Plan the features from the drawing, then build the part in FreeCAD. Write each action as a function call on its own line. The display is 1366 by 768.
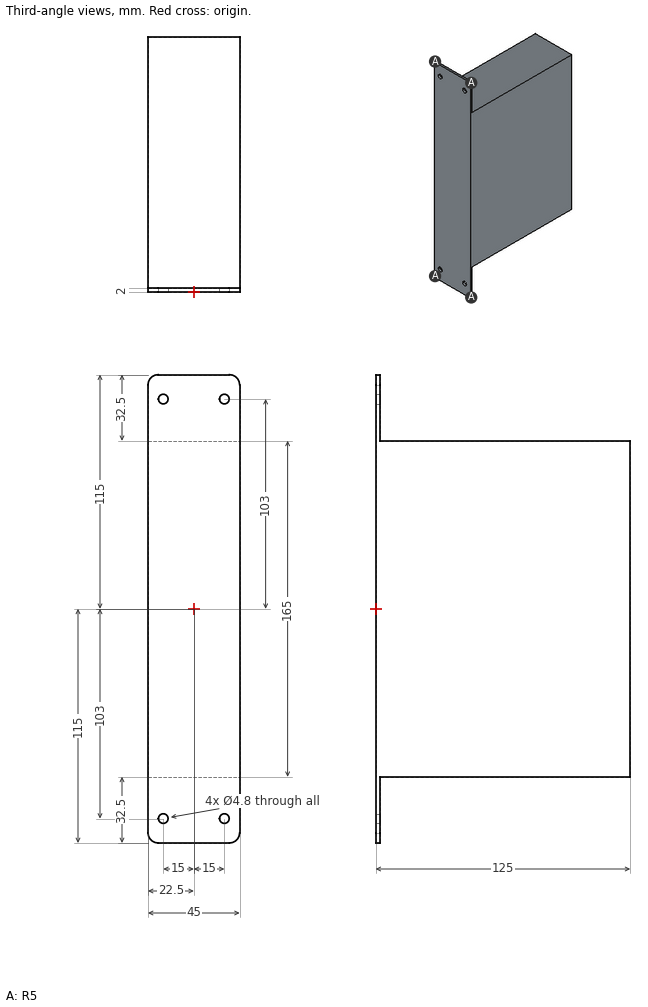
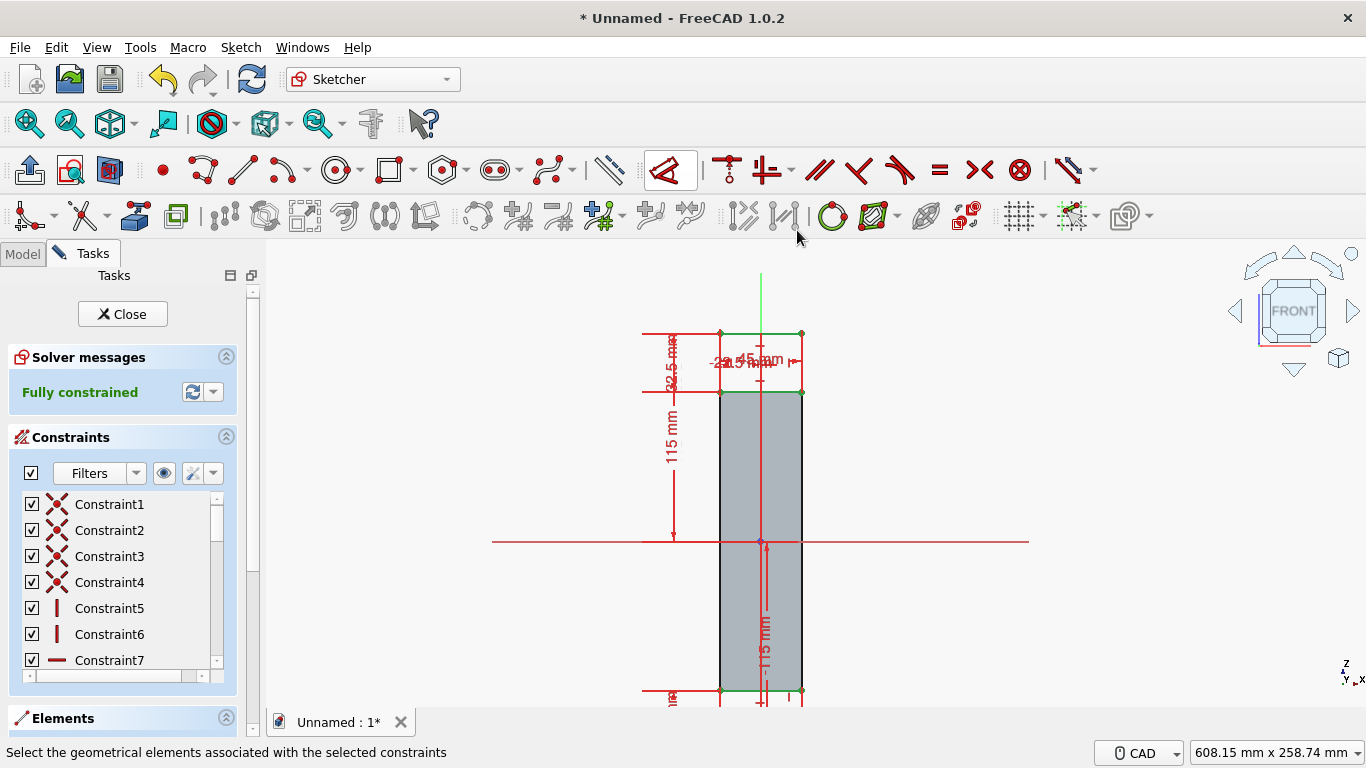
click(123, 314)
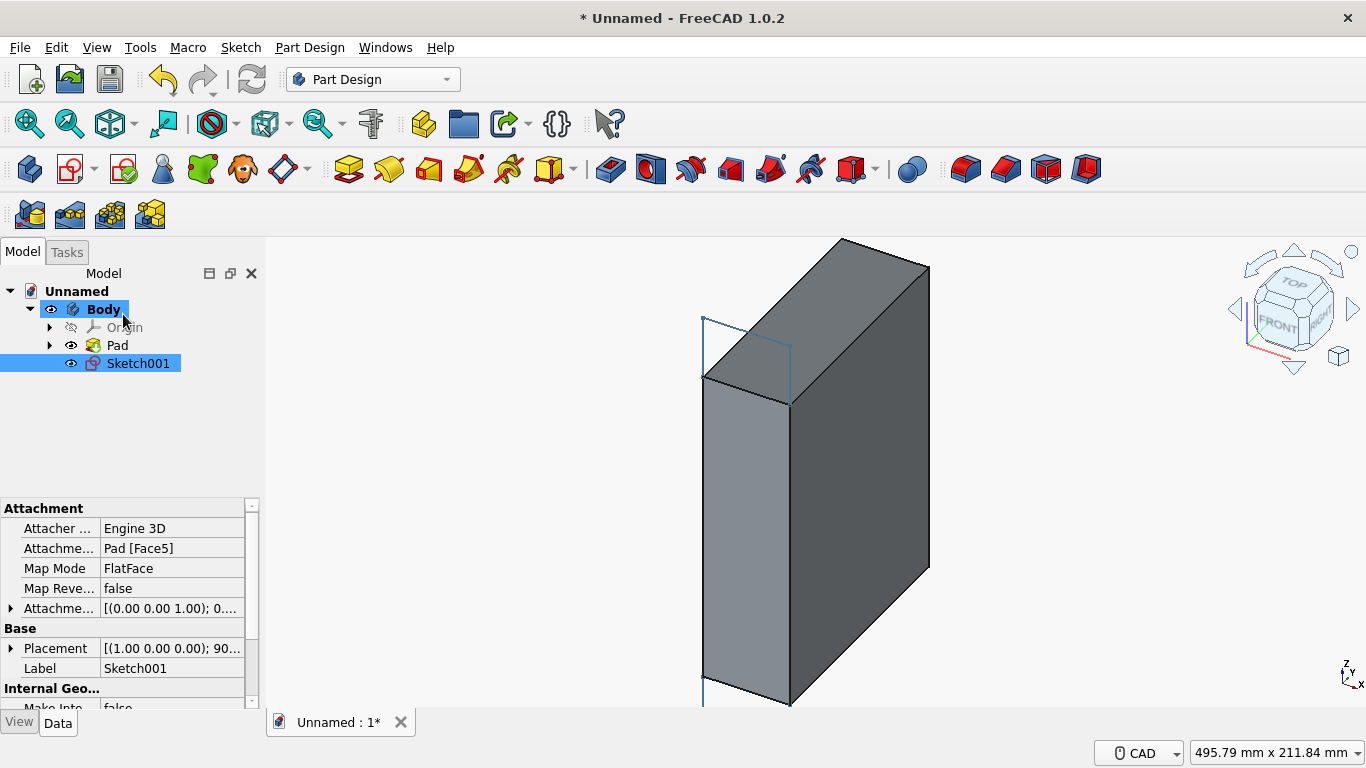
click(350, 170)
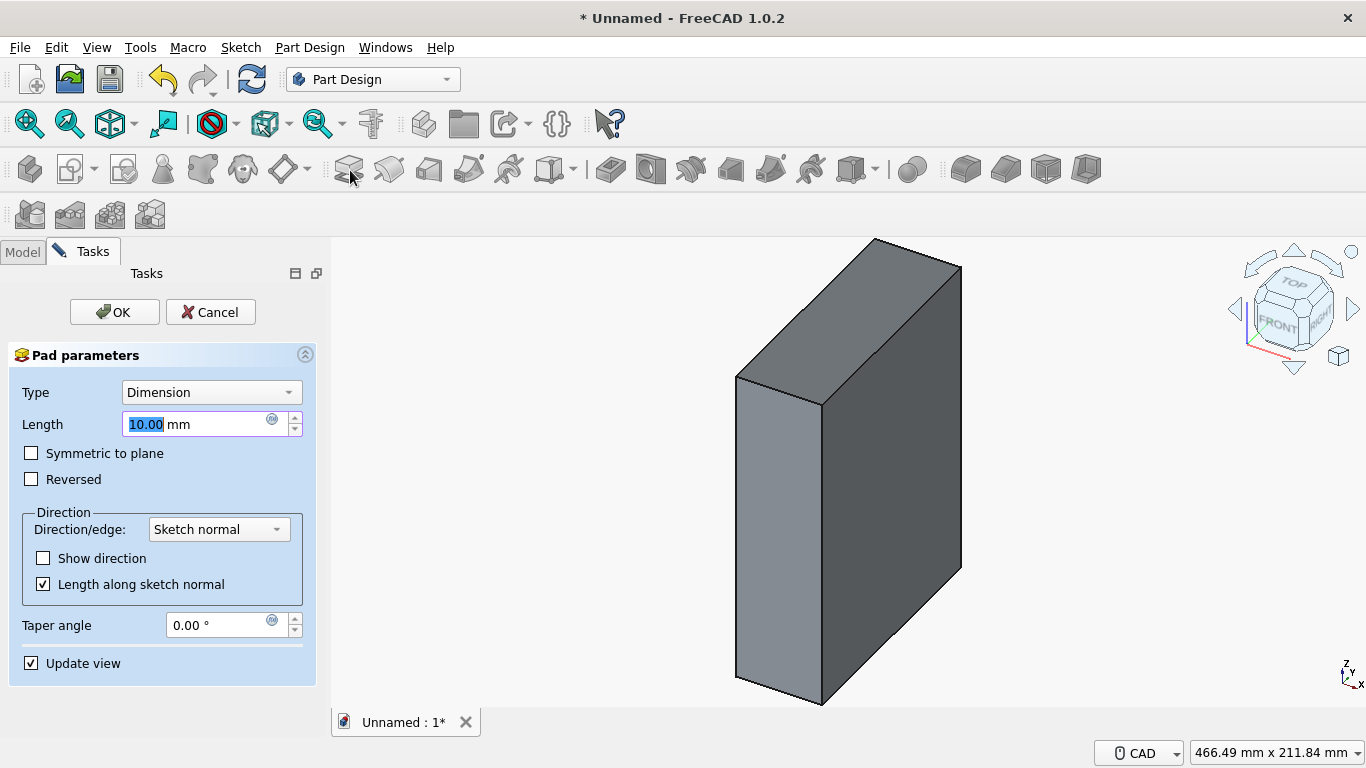
text(2)
key(Tab)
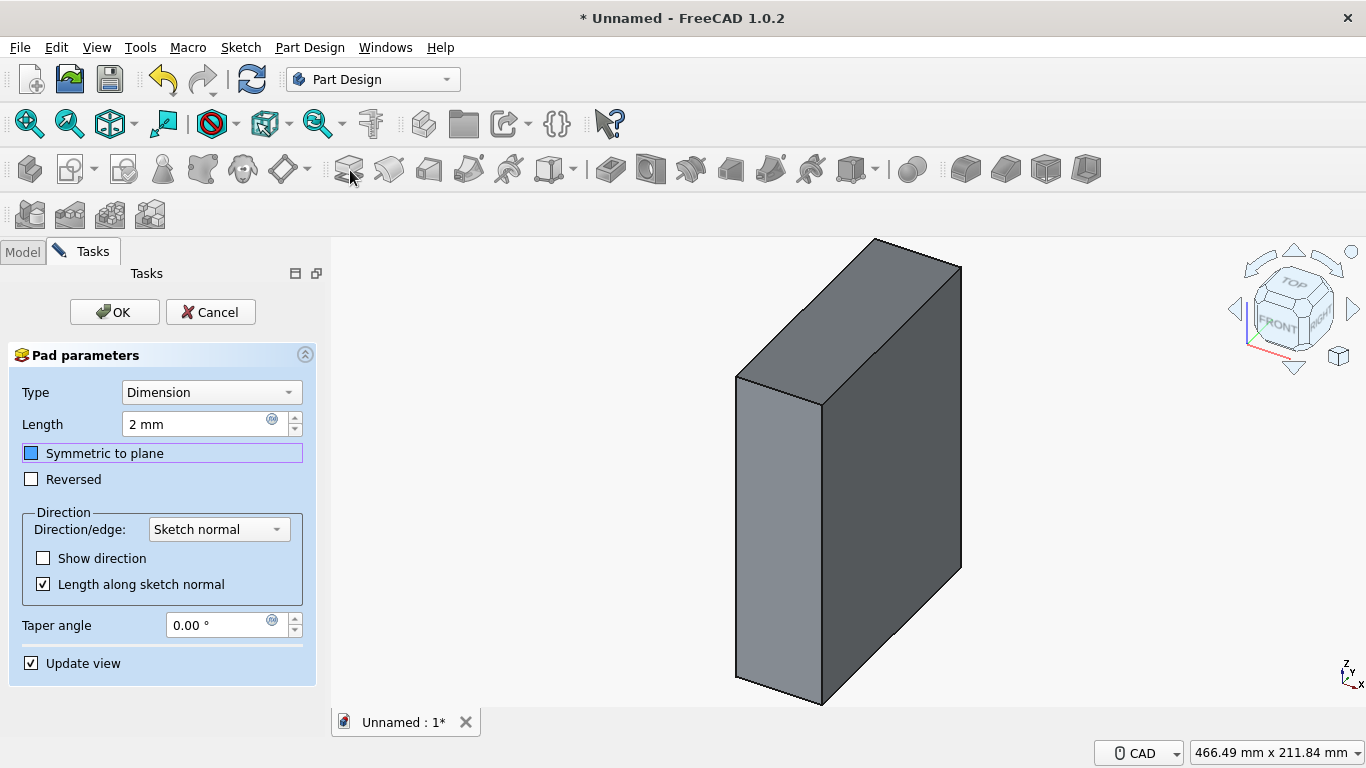
click(30, 479)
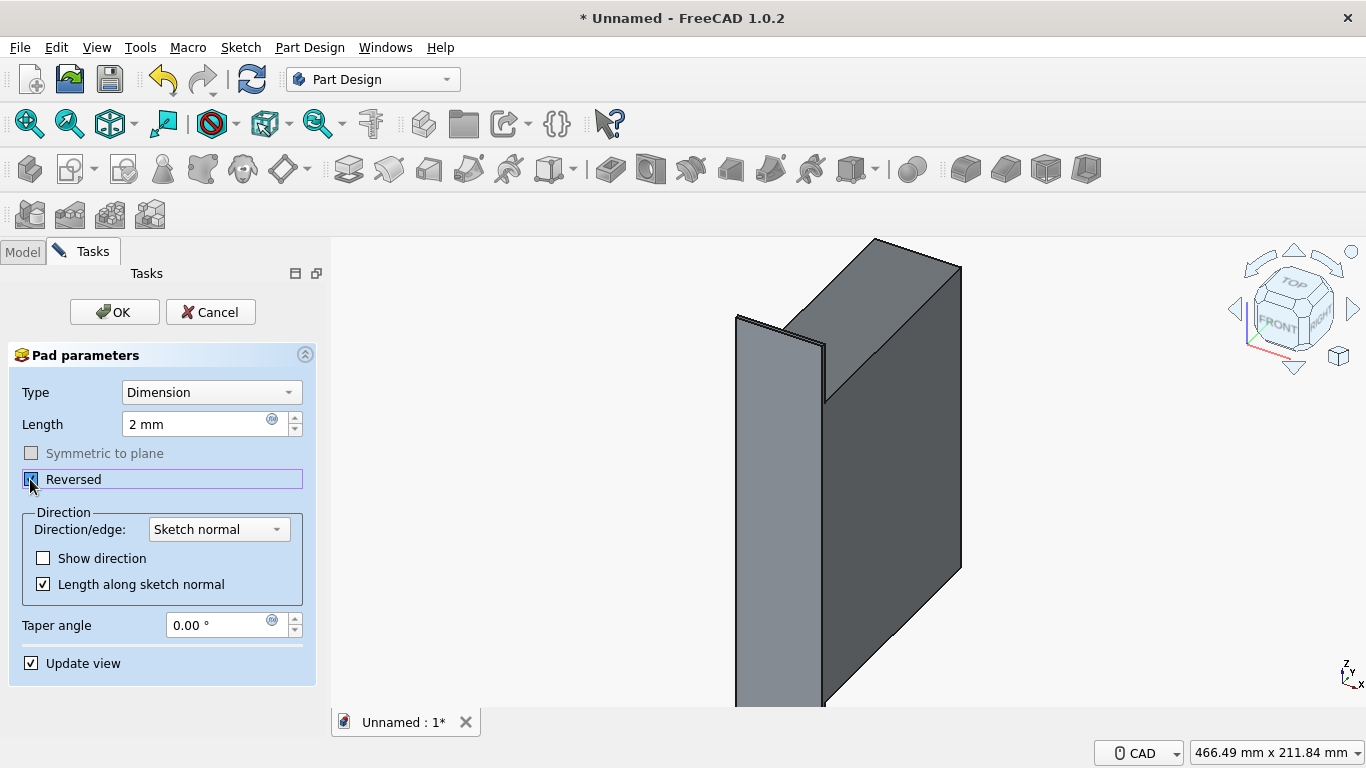
click(115, 312)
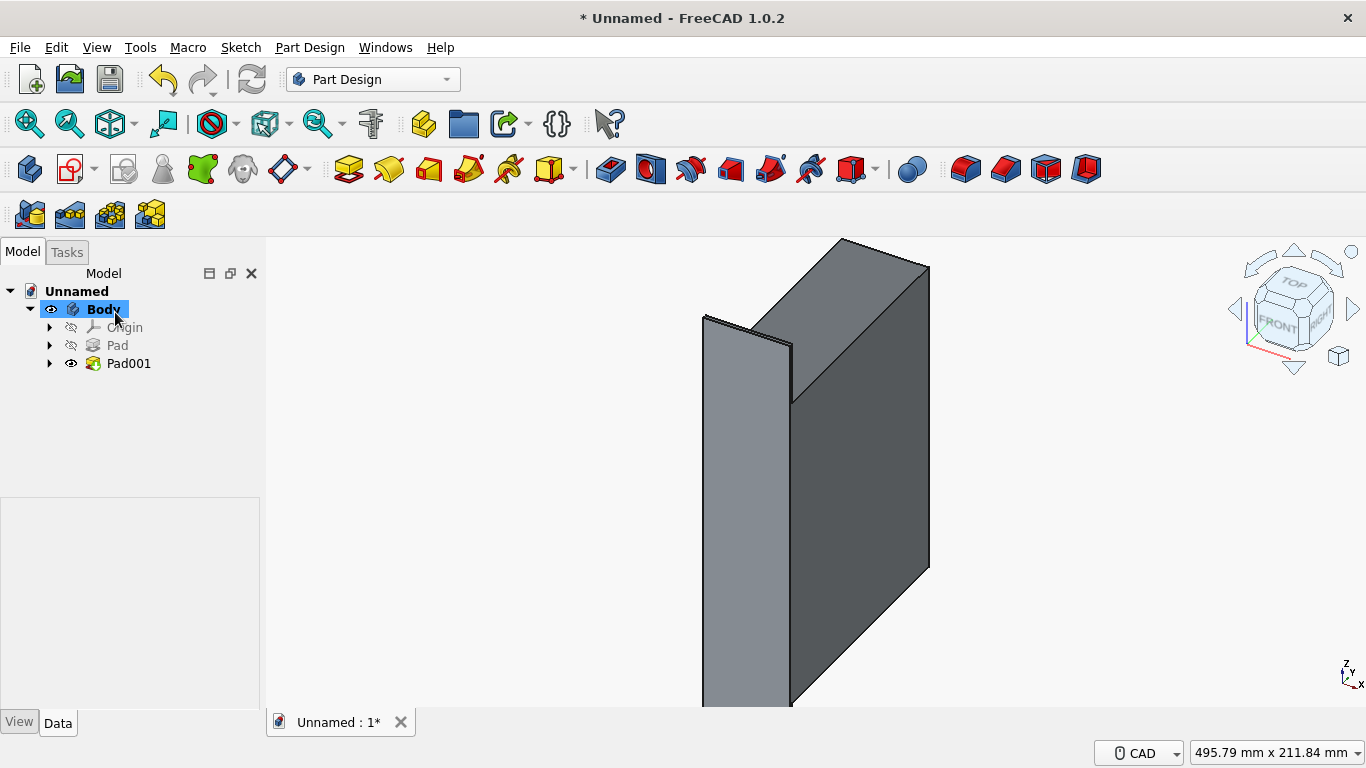
click(30, 124)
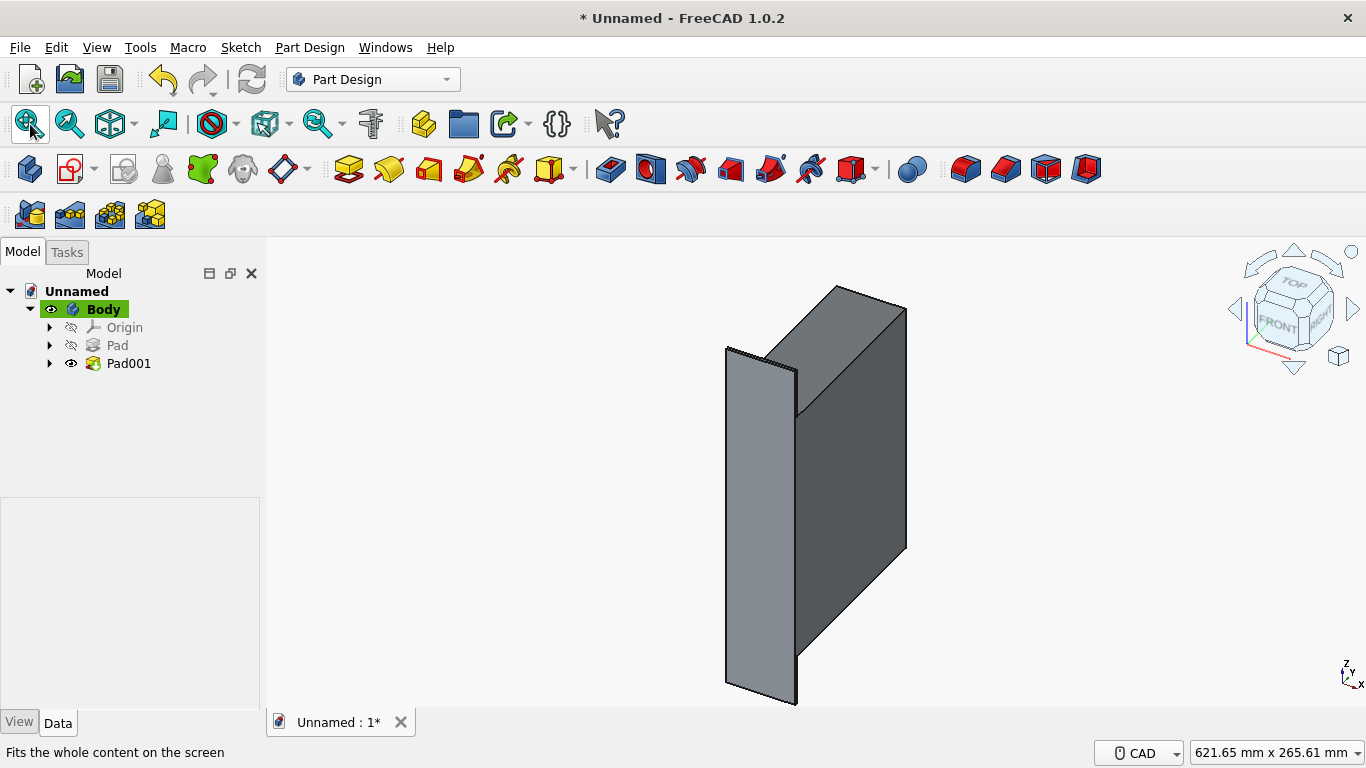
key(4)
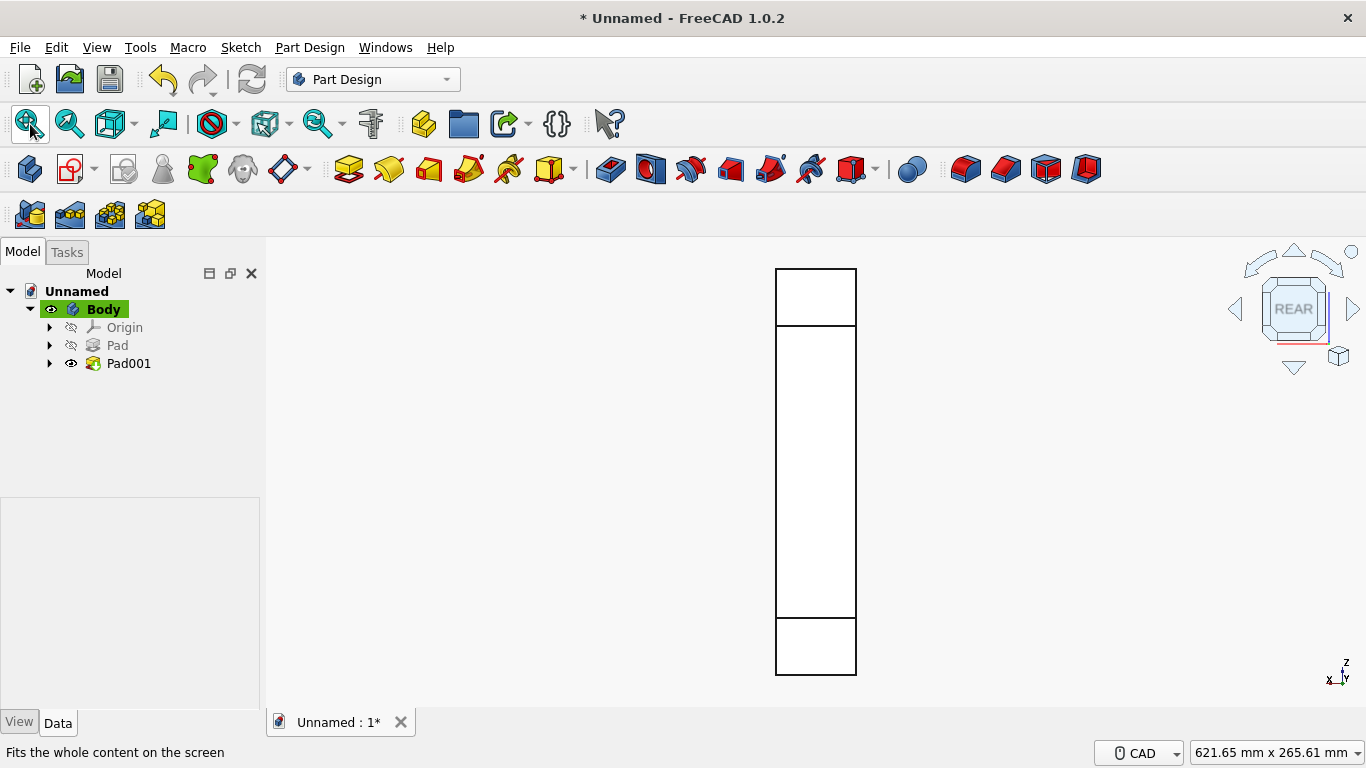
click(816, 296)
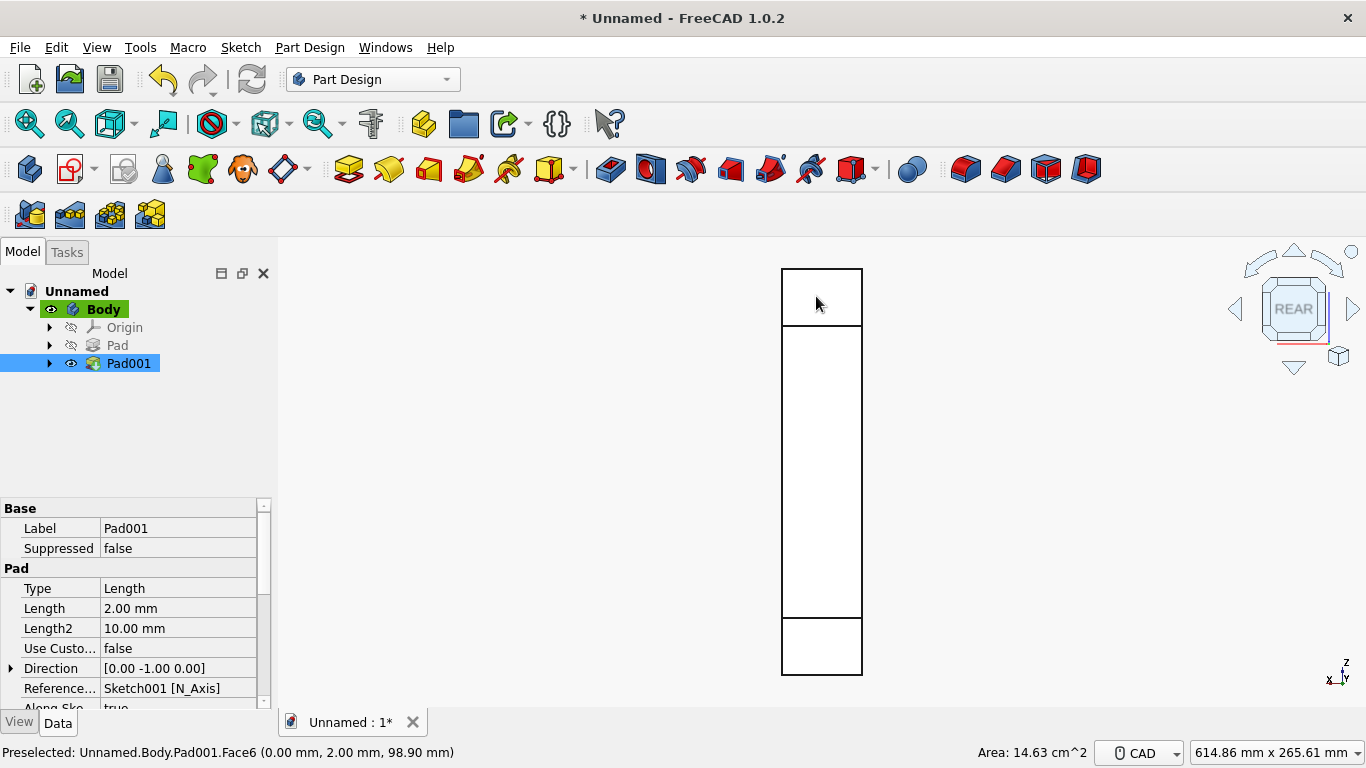
click(70, 170)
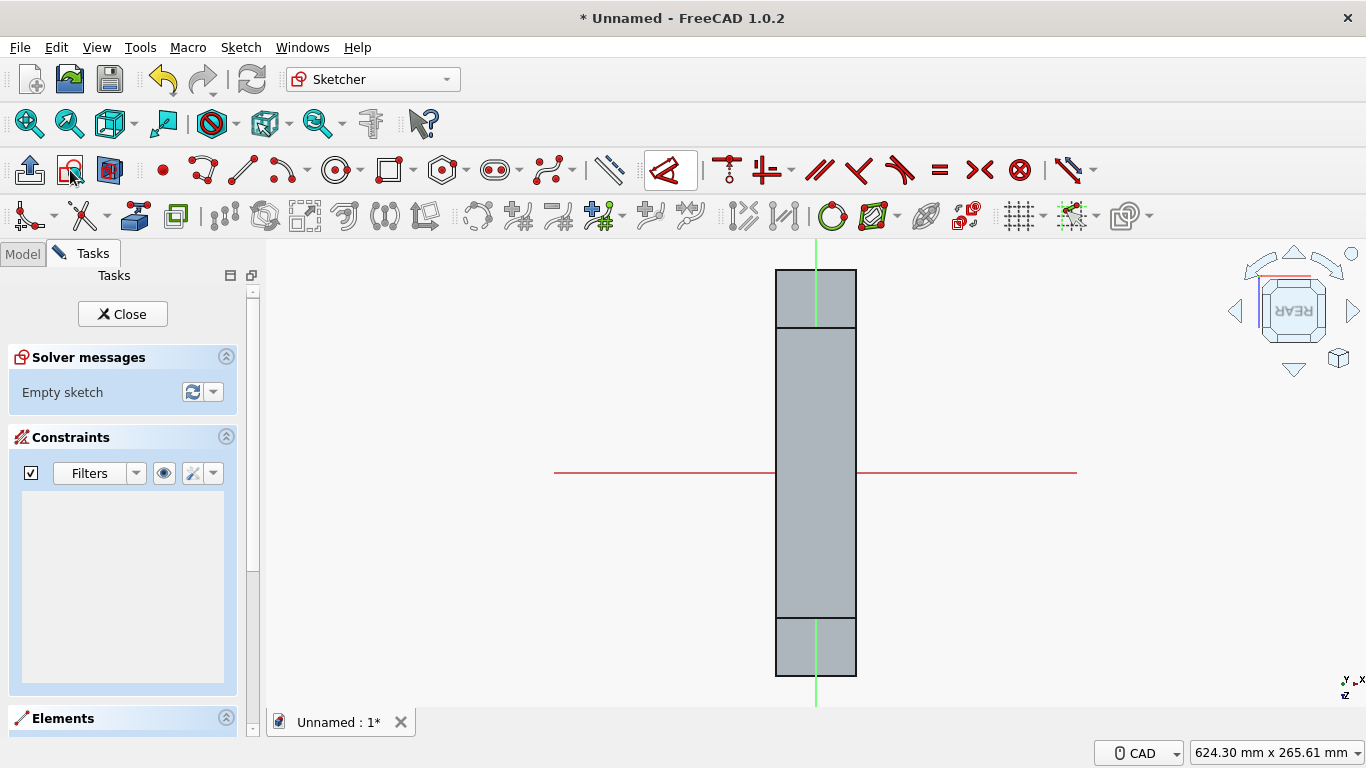
scroll(438, 473, down, 1)